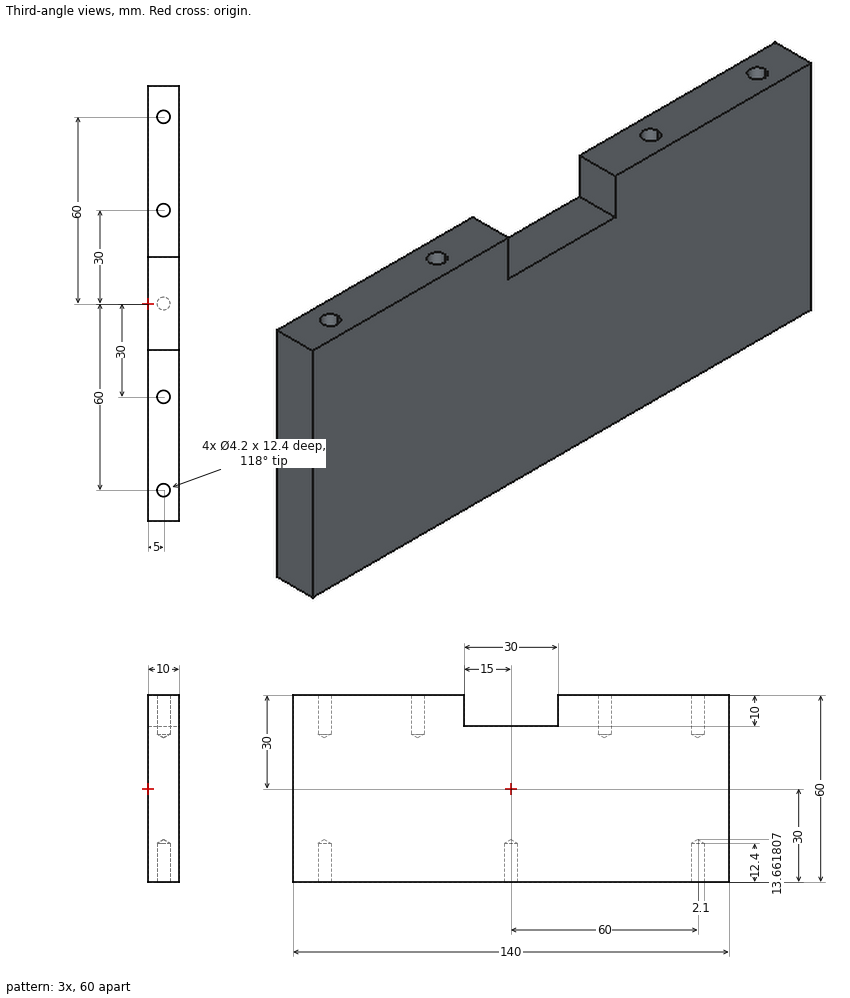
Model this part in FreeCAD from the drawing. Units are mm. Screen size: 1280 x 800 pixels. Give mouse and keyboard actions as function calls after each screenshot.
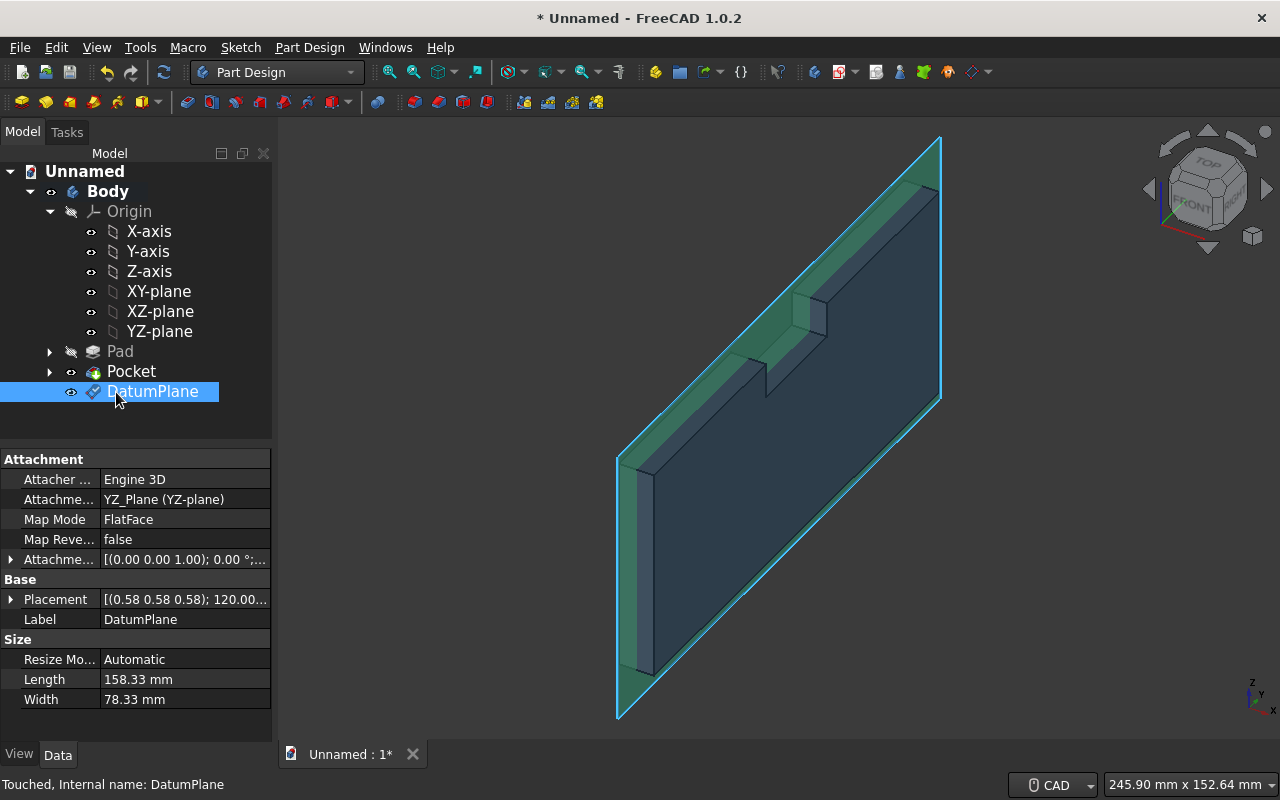
click(840, 72)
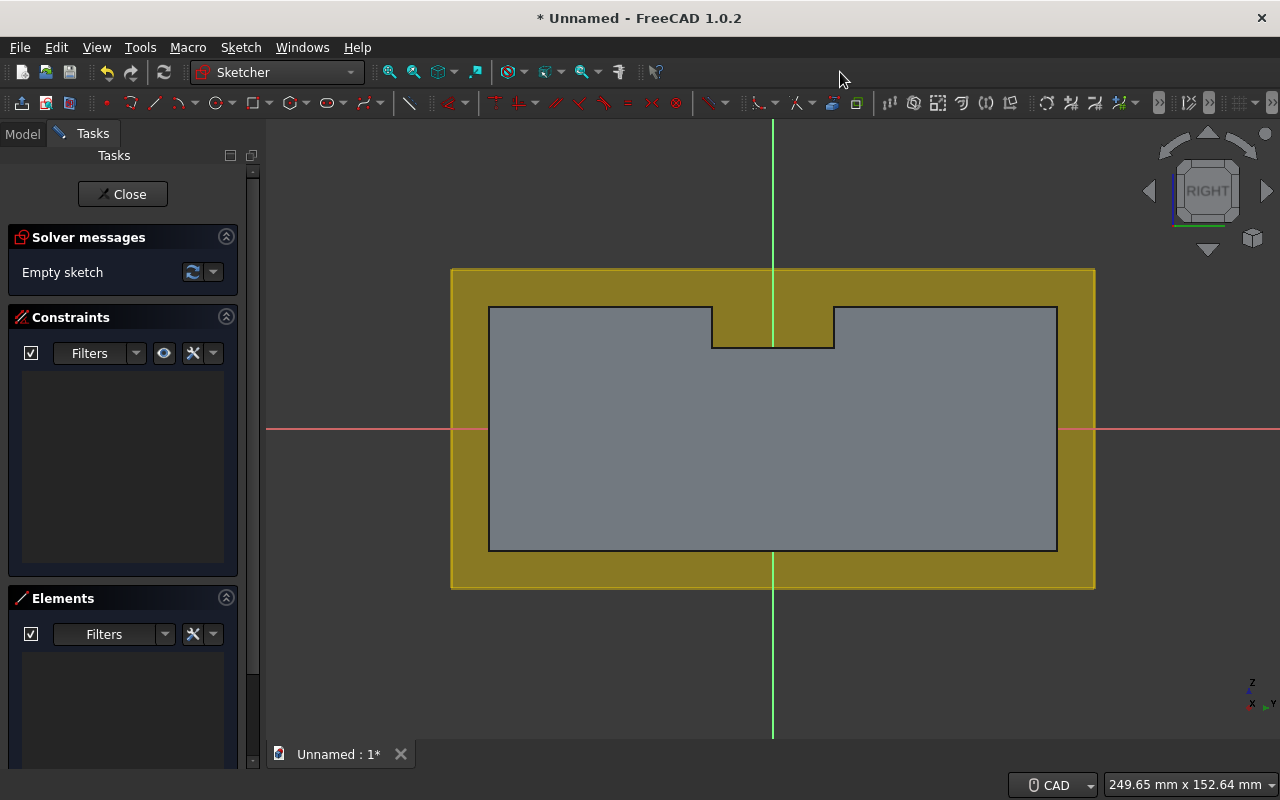
key(q)
key(s)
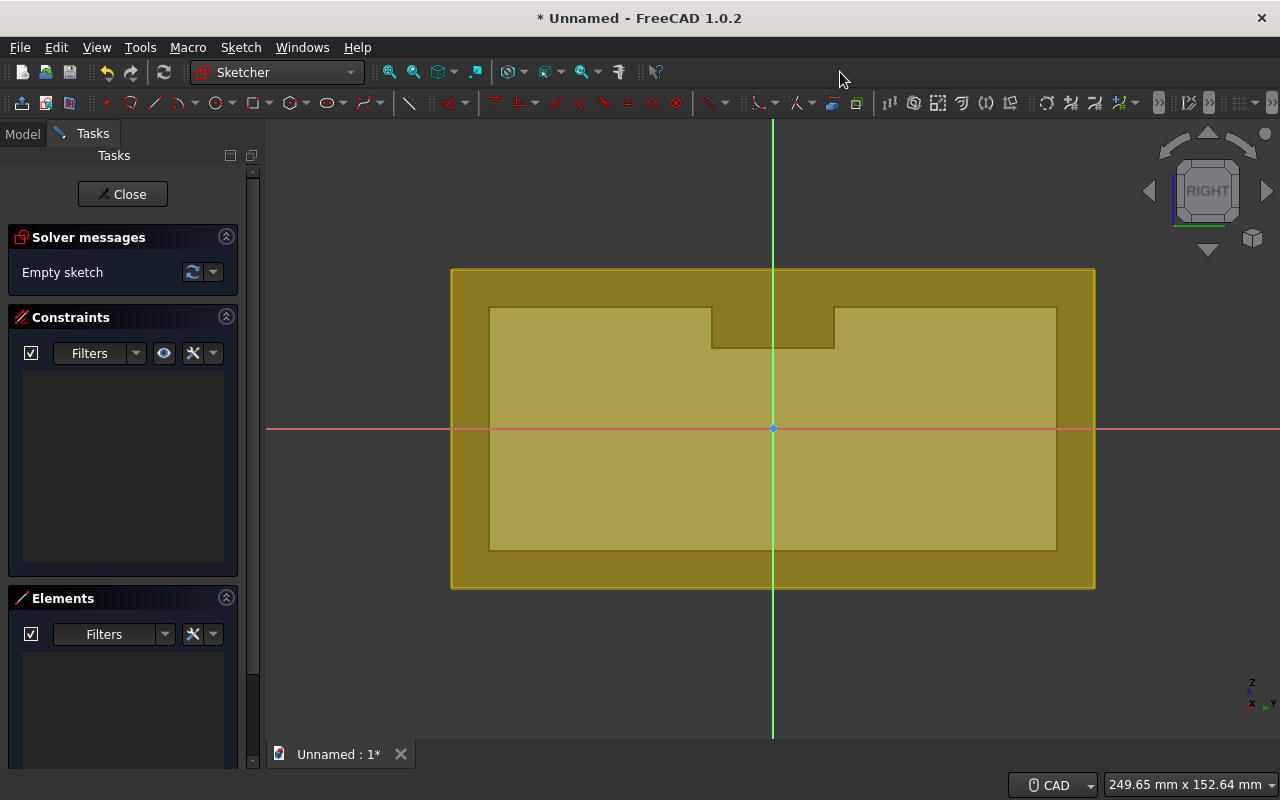
scroll(1101, 533, up, 8)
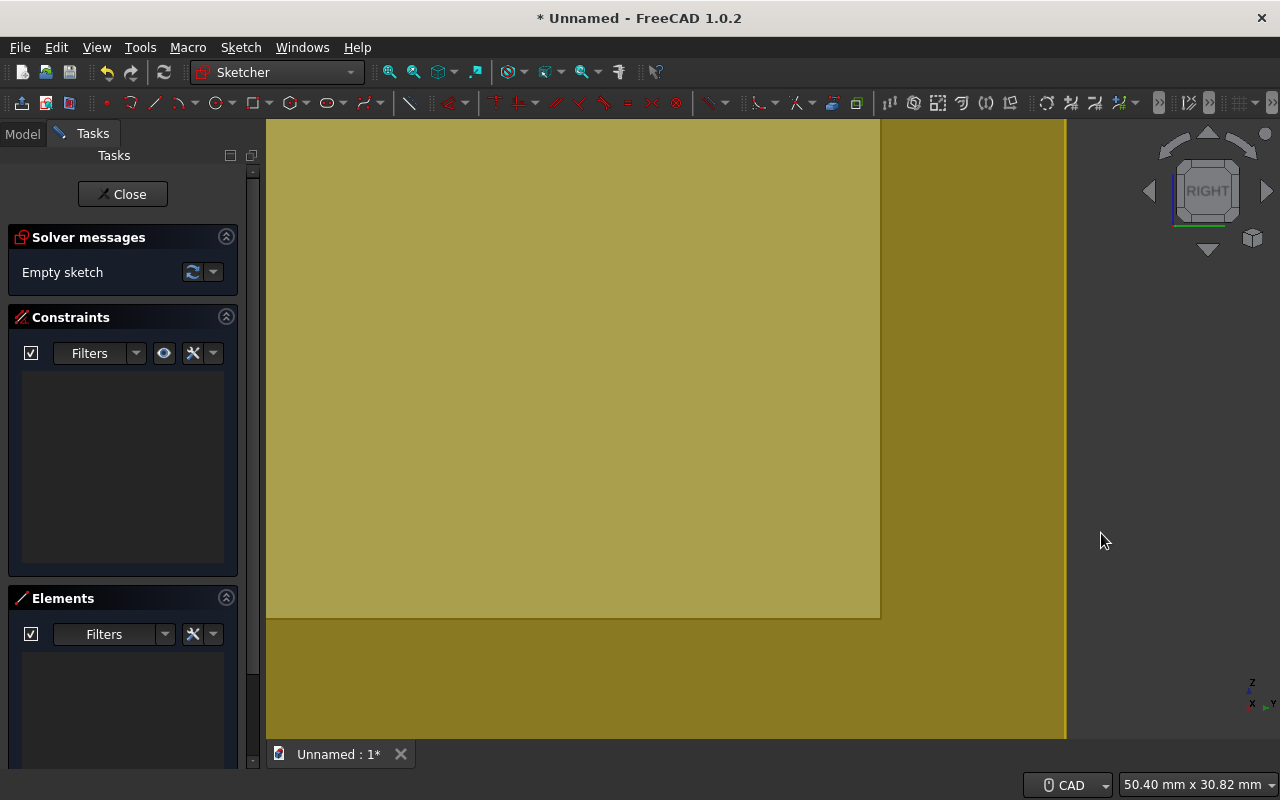
key(g)
key(m)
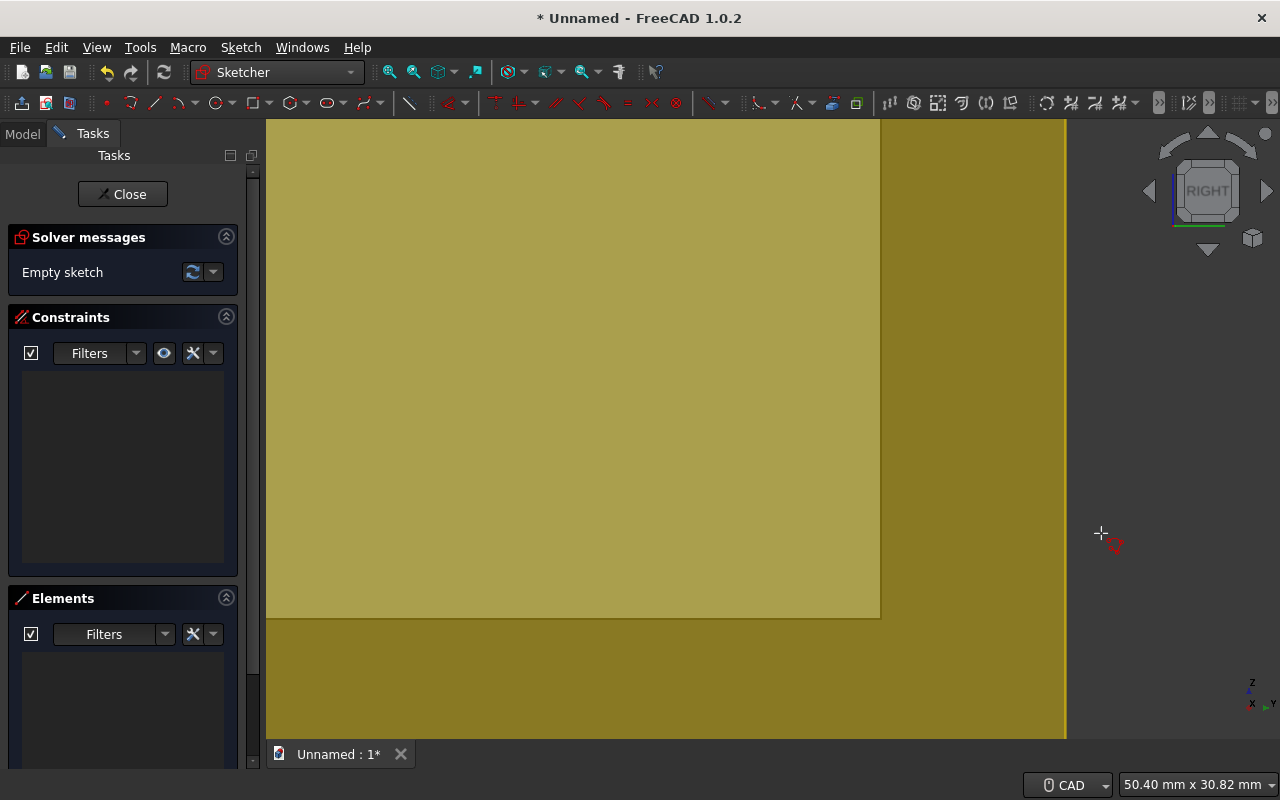
click(680, 344)
click(680, 619)
click(722, 619)
click(722, 369)
click(680, 345)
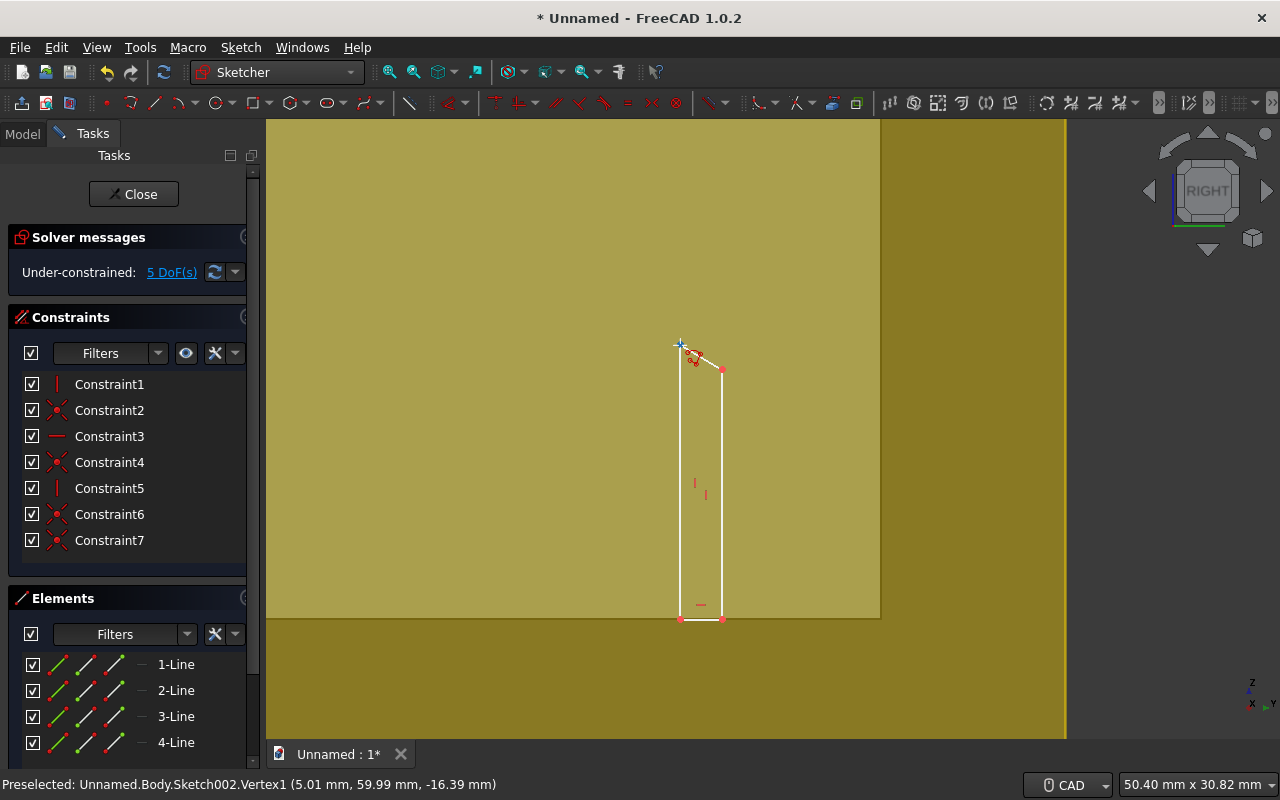
key(g)
key(l)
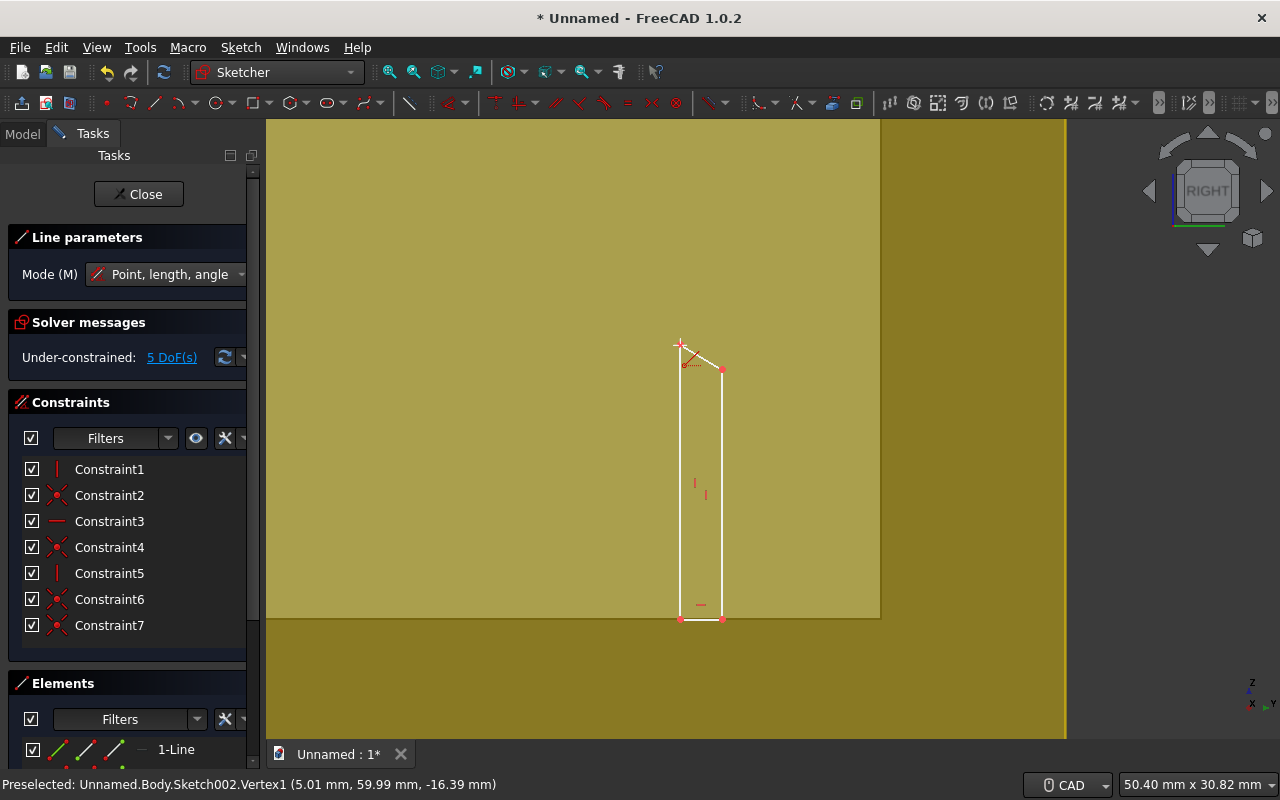
click(680, 316)
click(680, 234)
key(Escape)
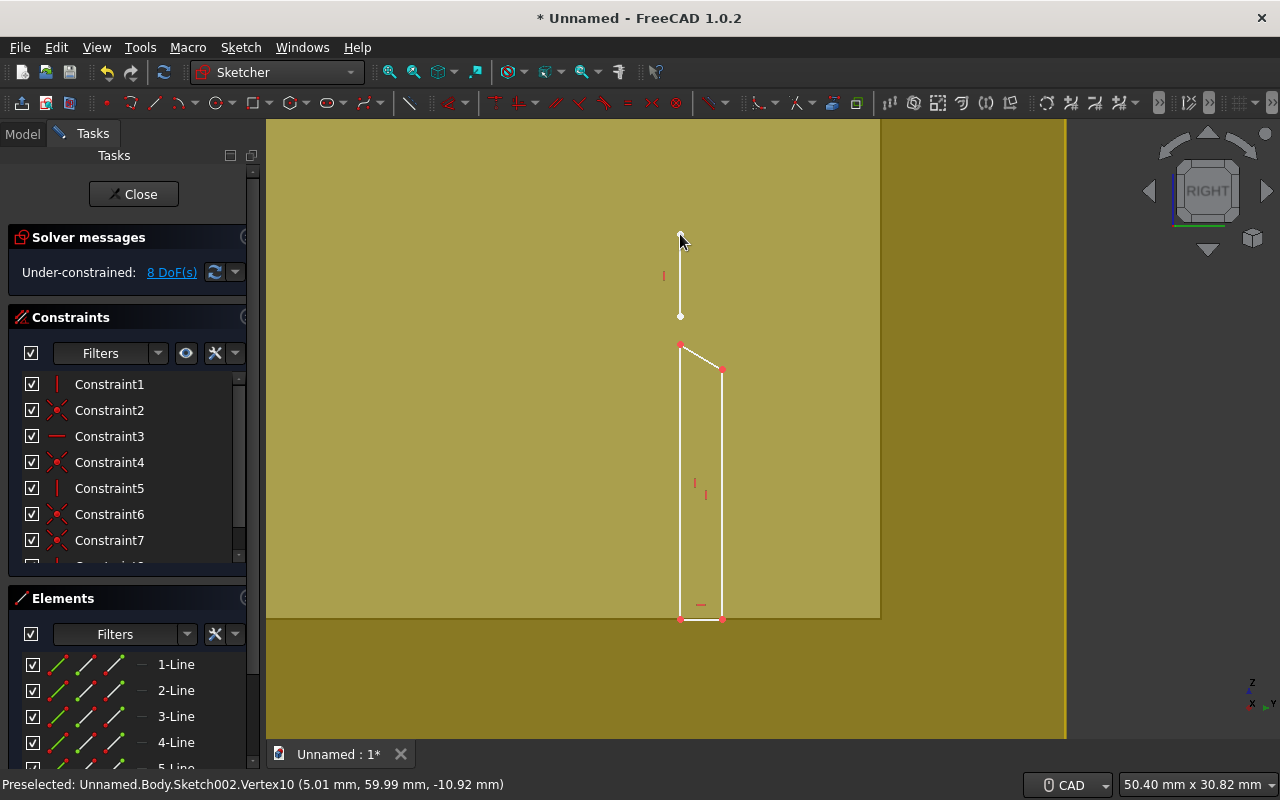
click(680, 292)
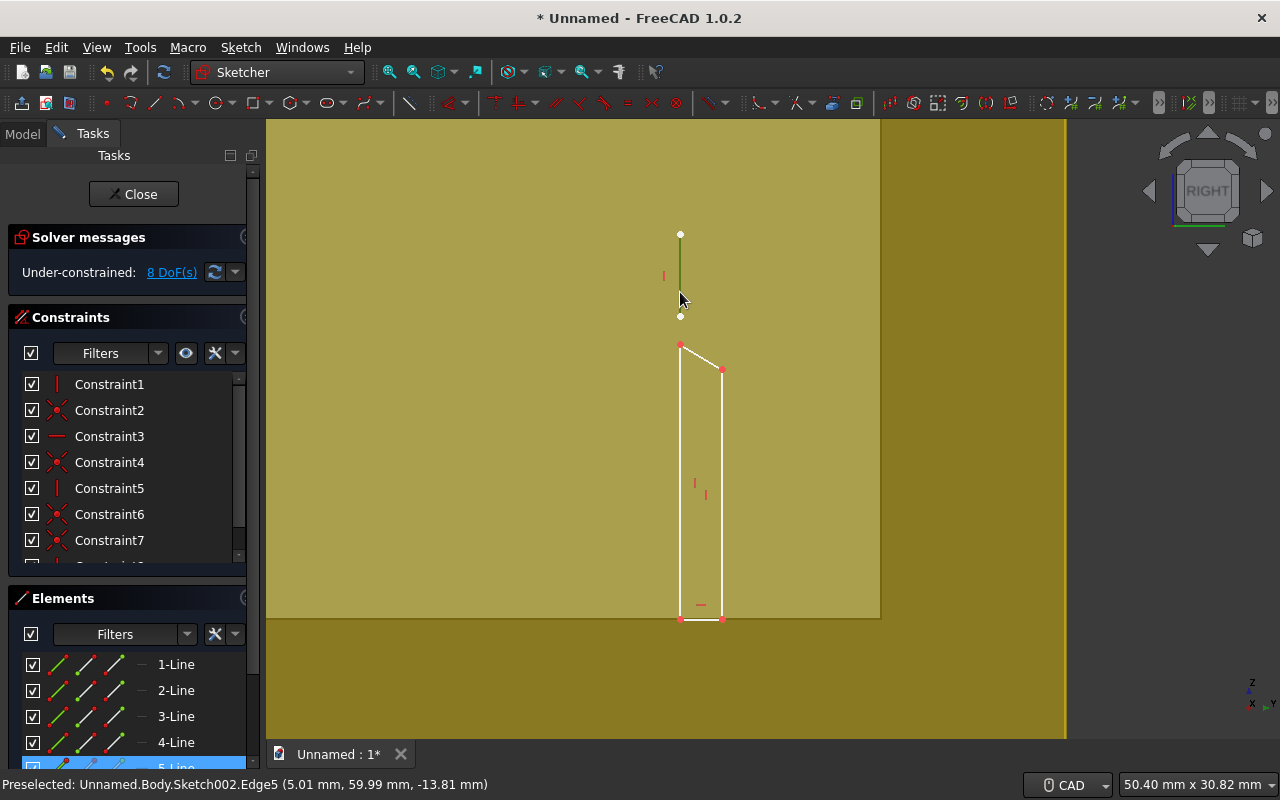
key(g)
key(n)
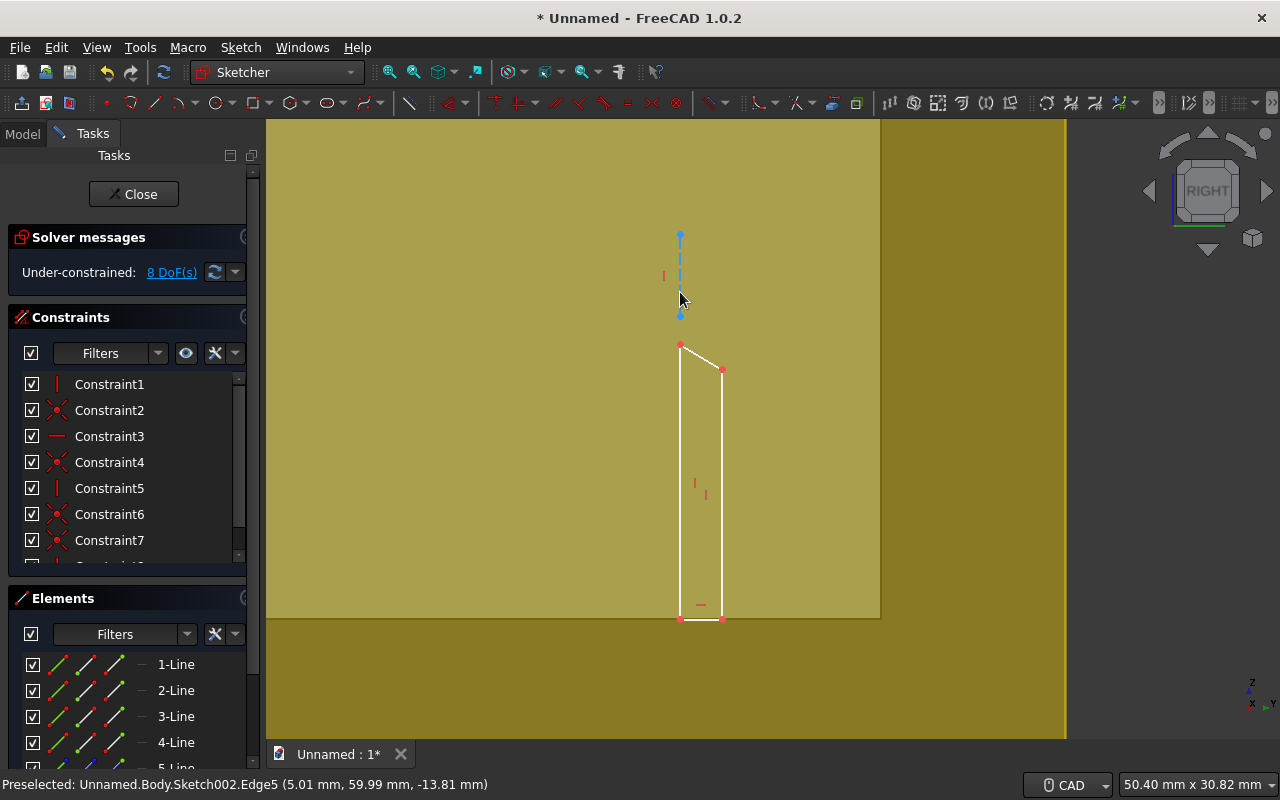
key(d)